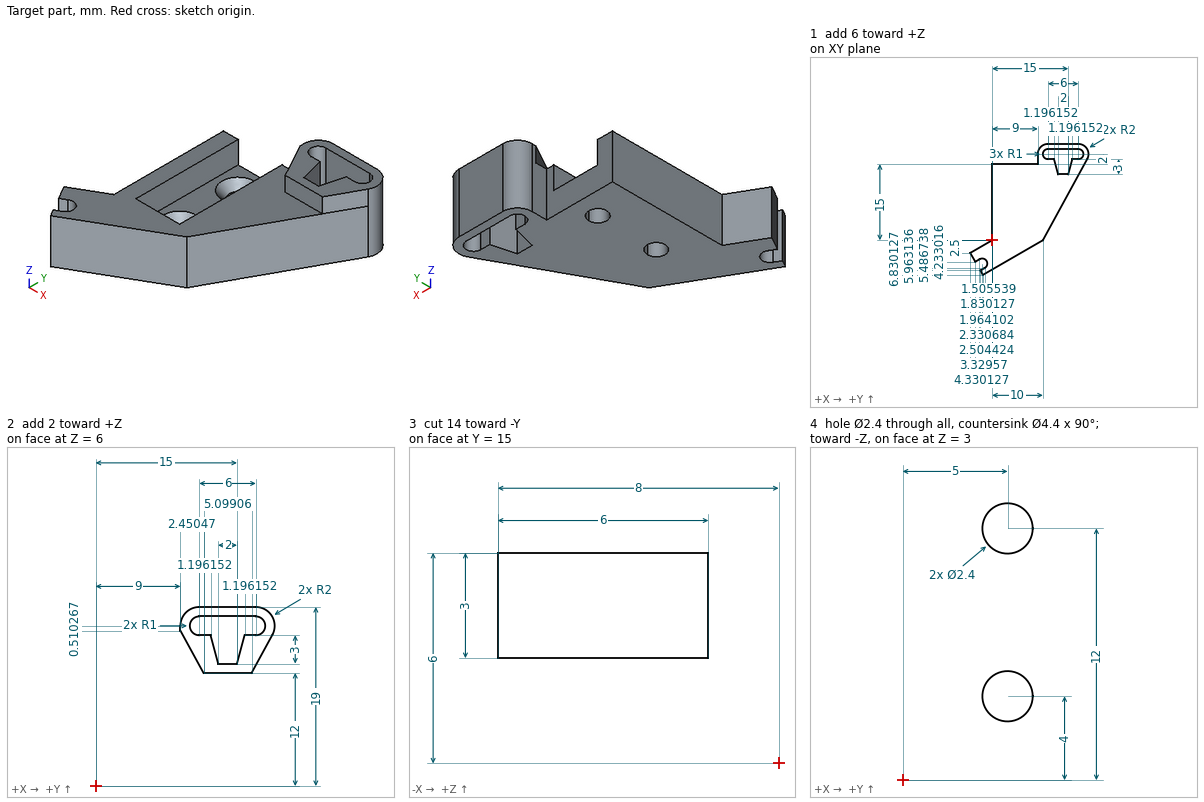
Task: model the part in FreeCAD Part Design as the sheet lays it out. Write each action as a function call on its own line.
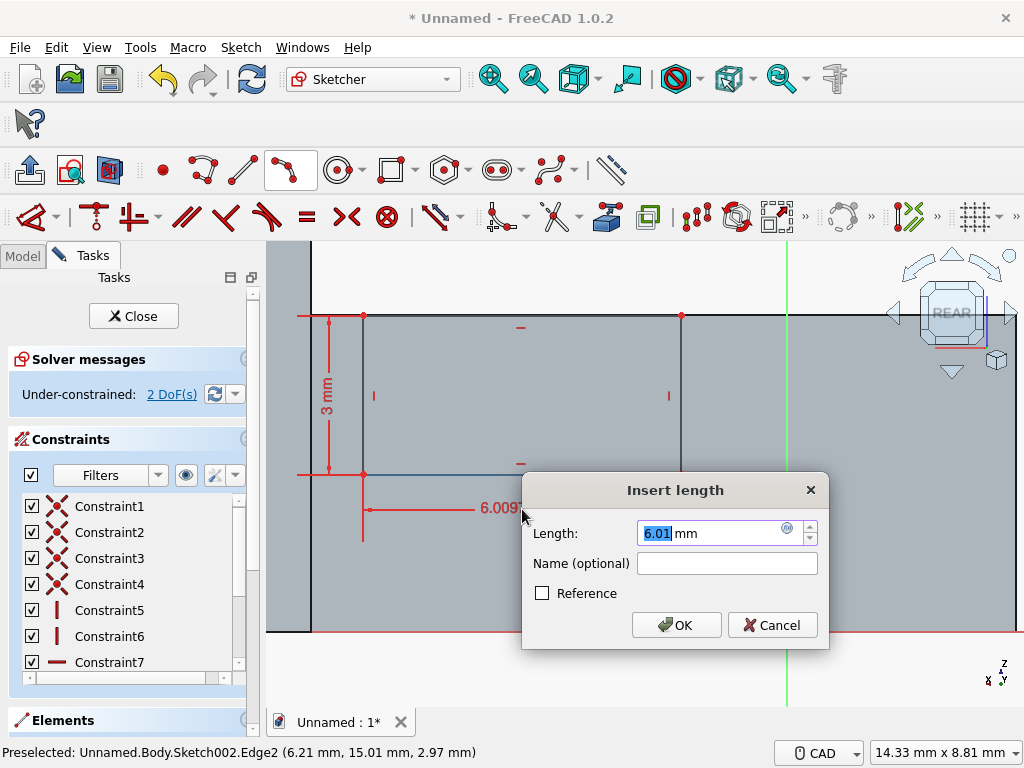
text(6)
key(Return)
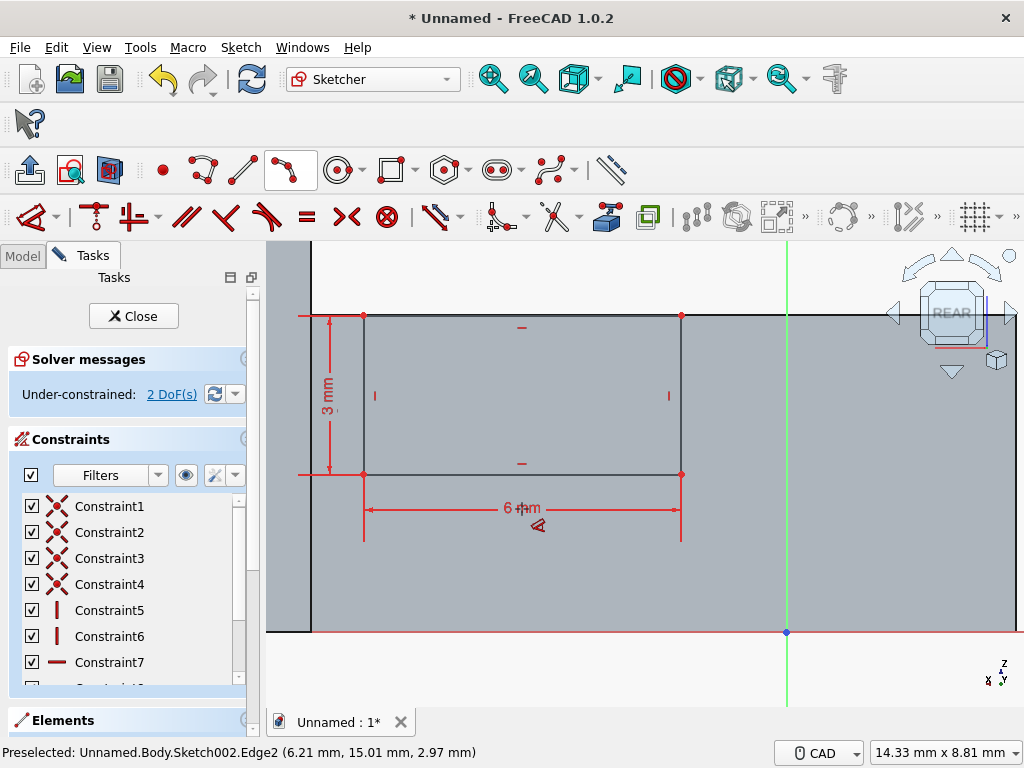
click(364, 316)
click(575, 666)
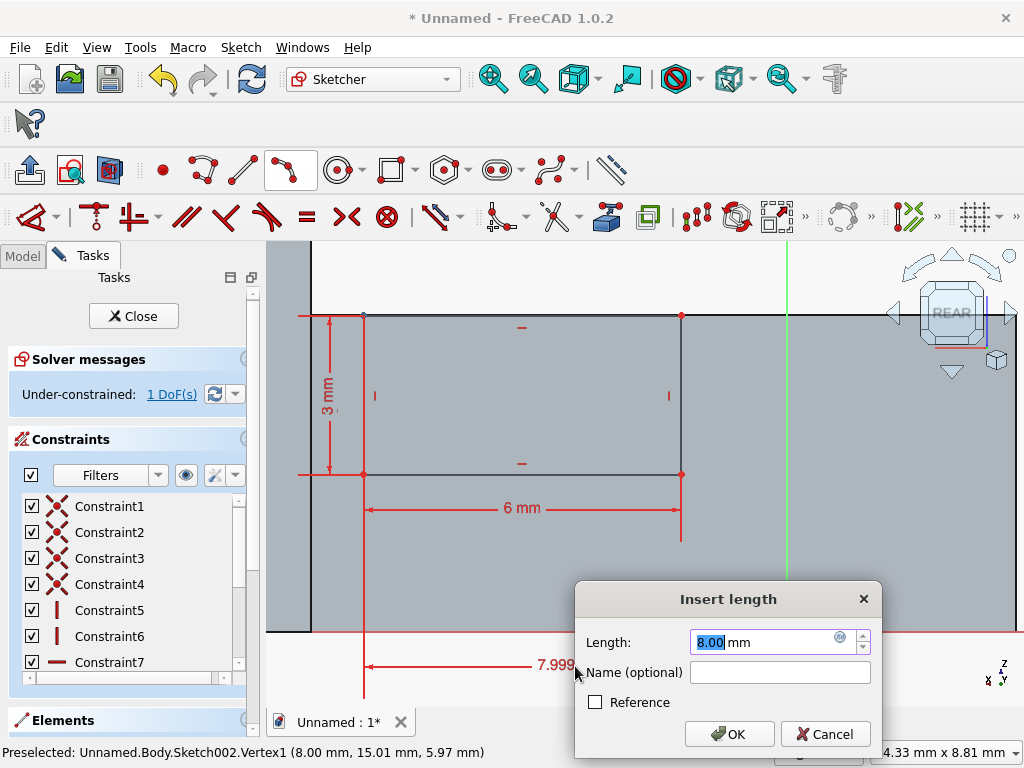
text(8)
key(Return)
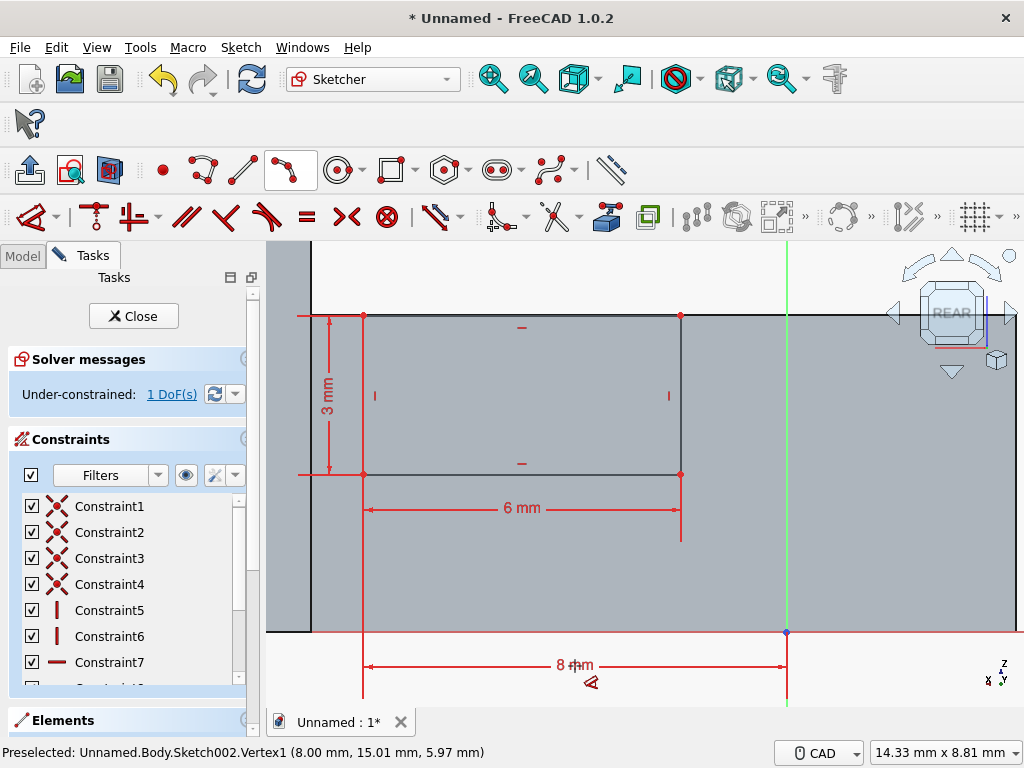
click(363, 316)
click(821, 474)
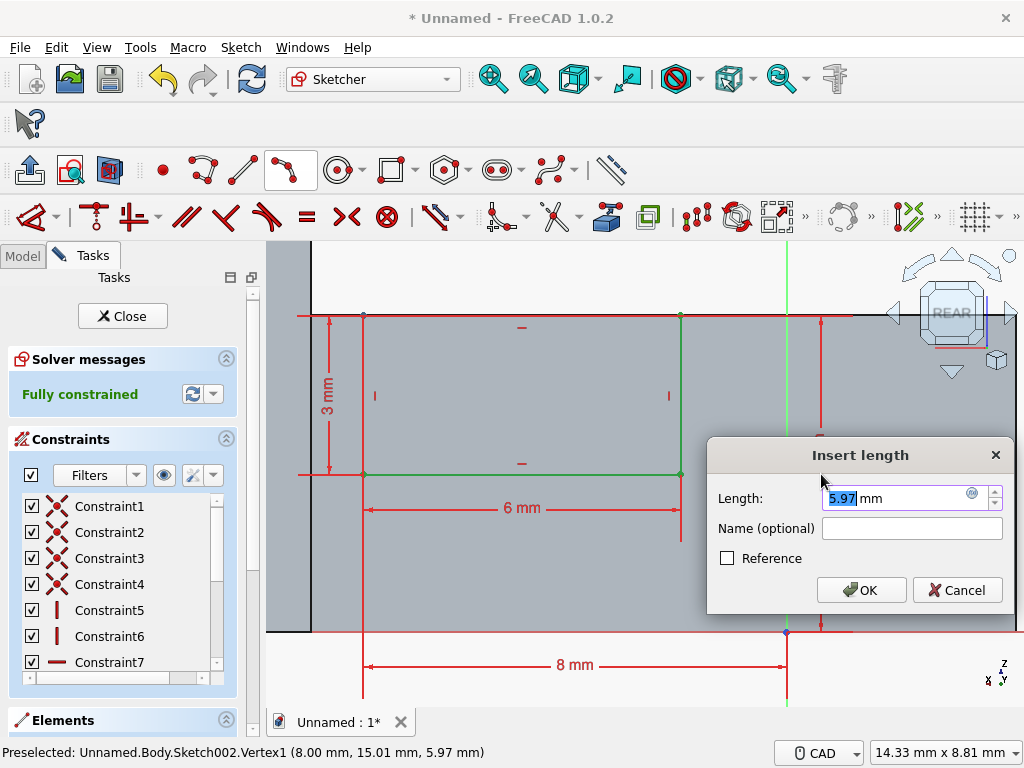
text(6)
key(Return)
key(Escape)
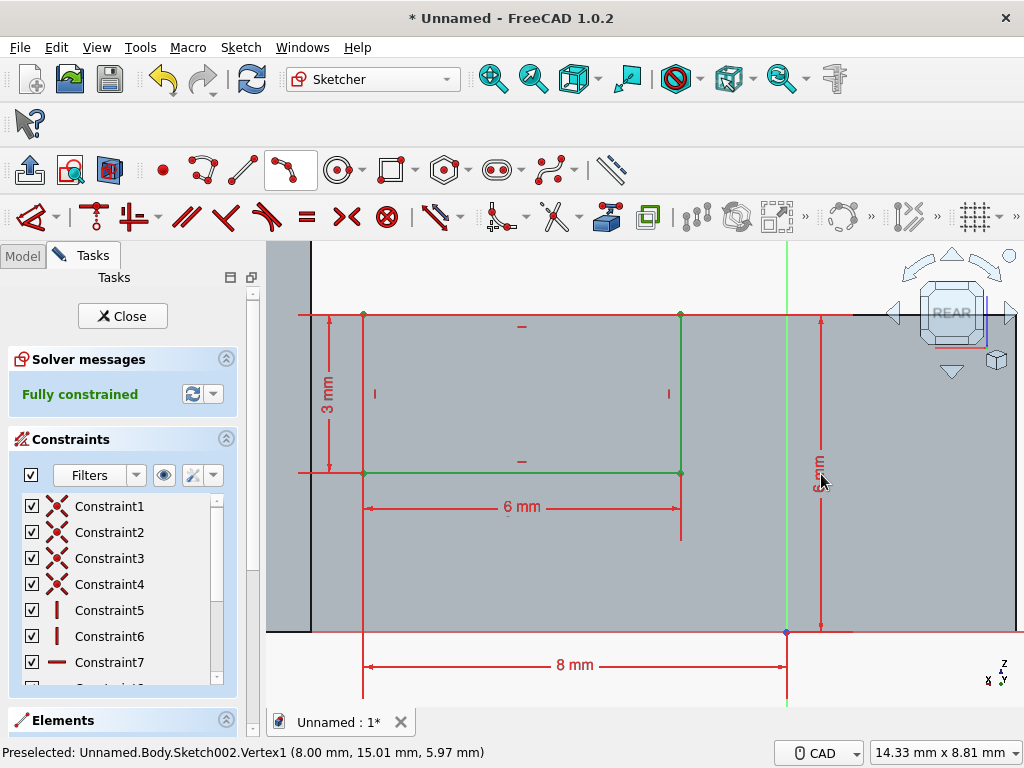
click(123, 316)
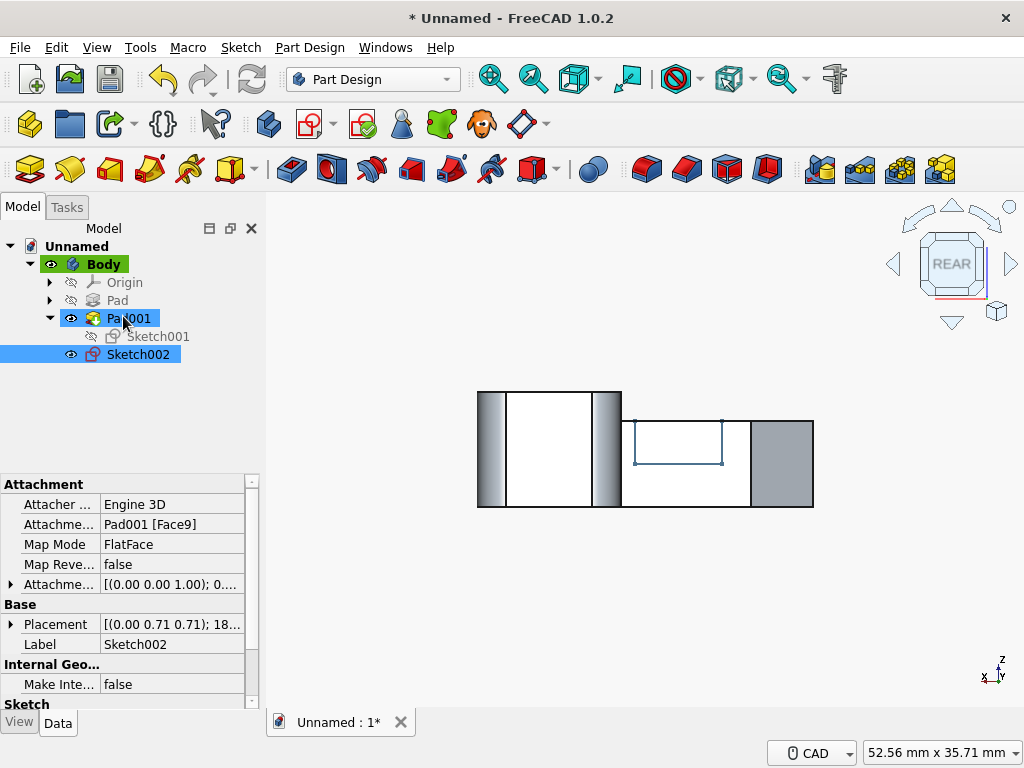
click(292, 170)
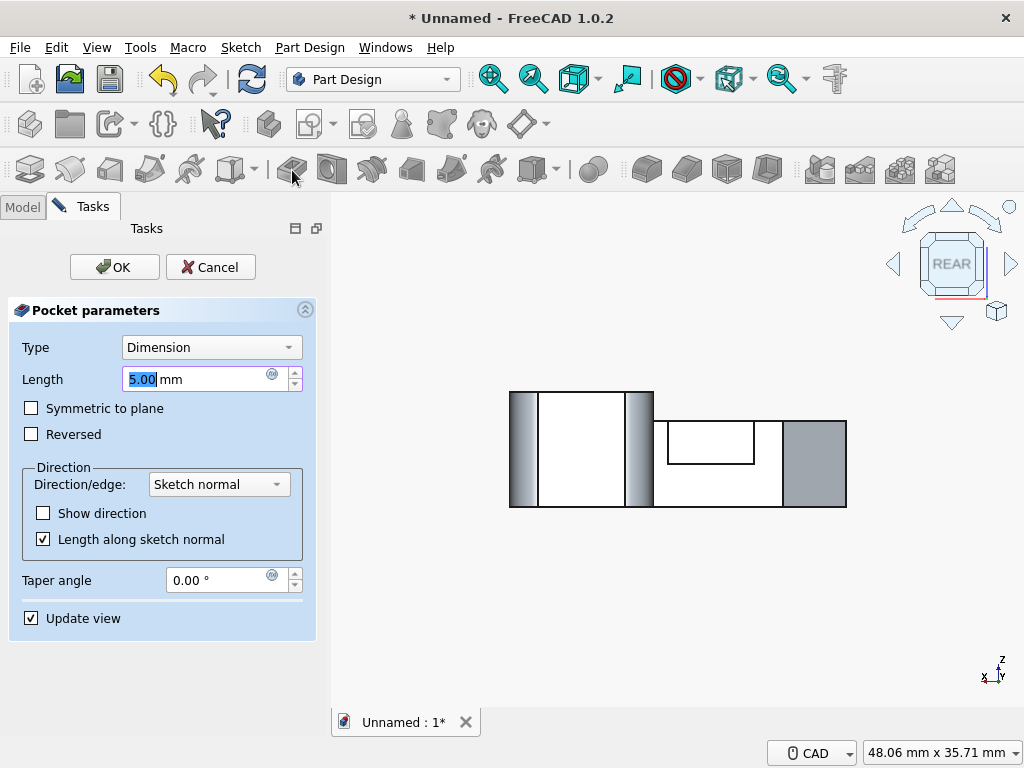
text(14)
key(Tab)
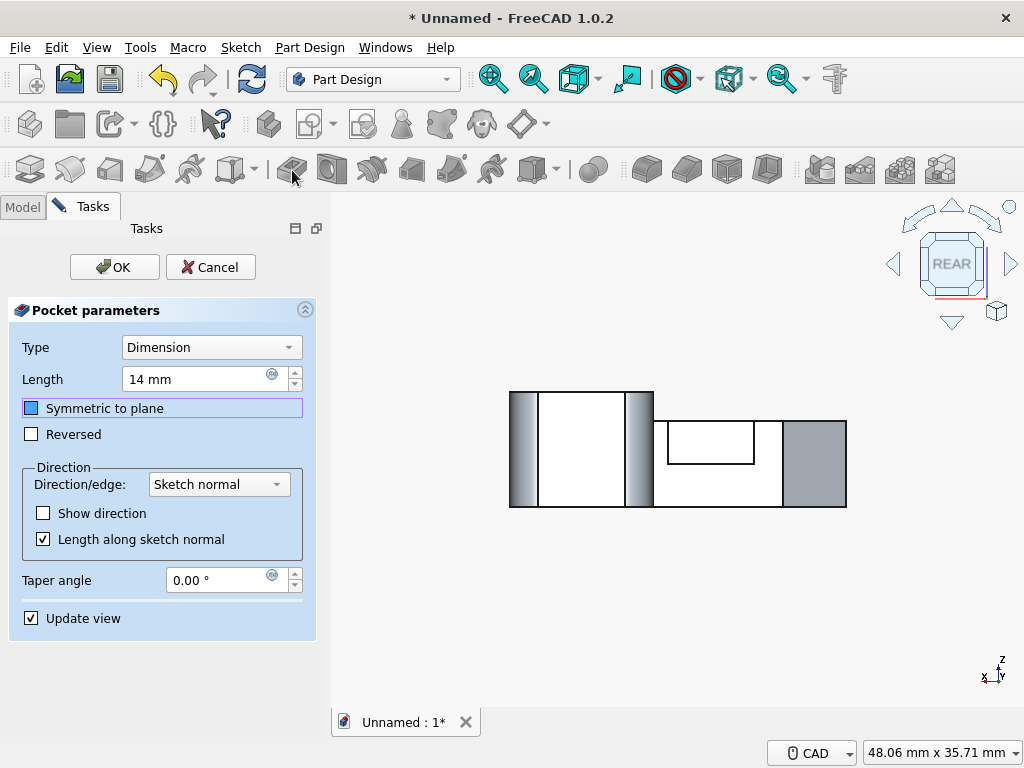
click(115, 267)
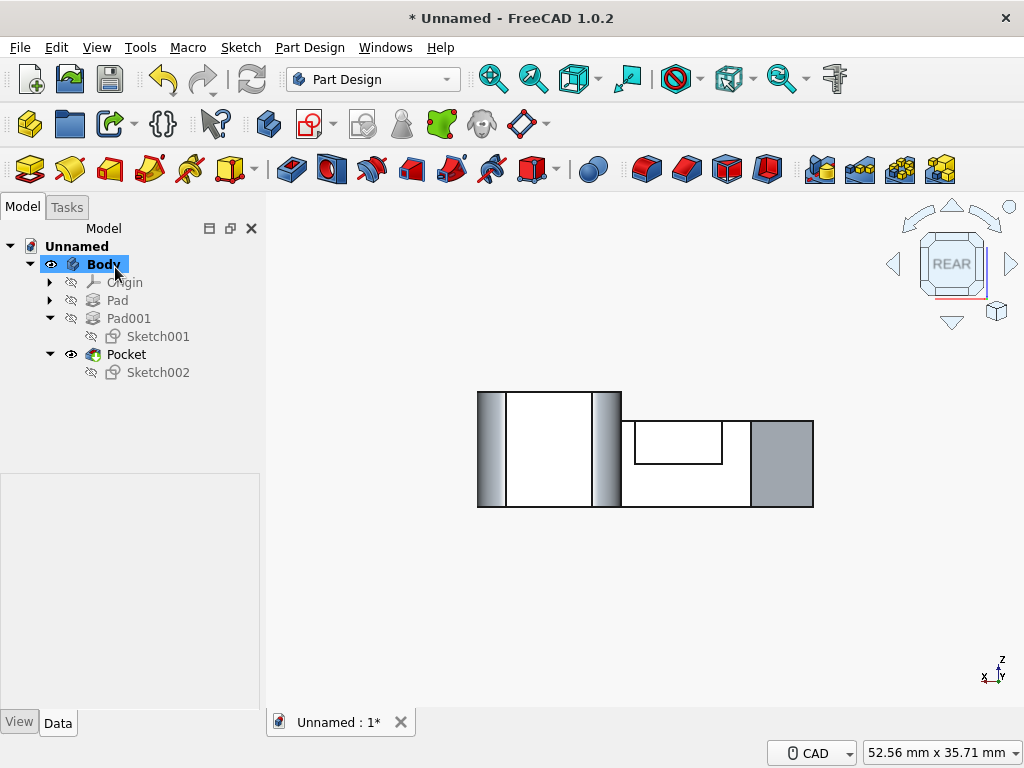
key(v)
key(f)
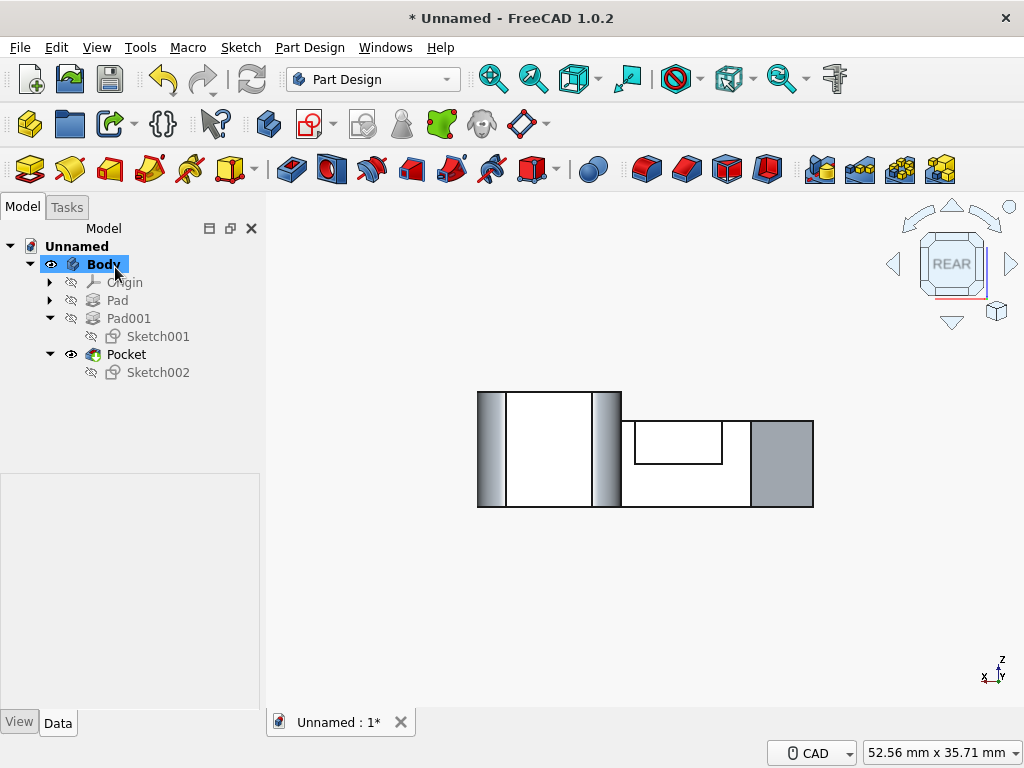
key(0)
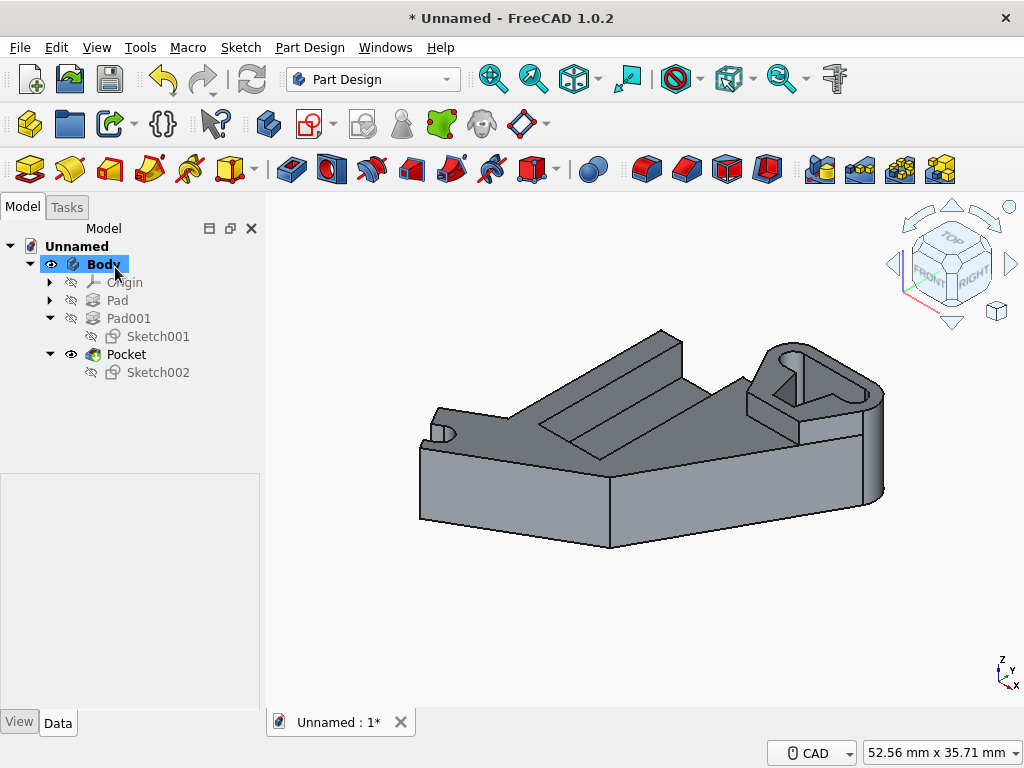
key(2)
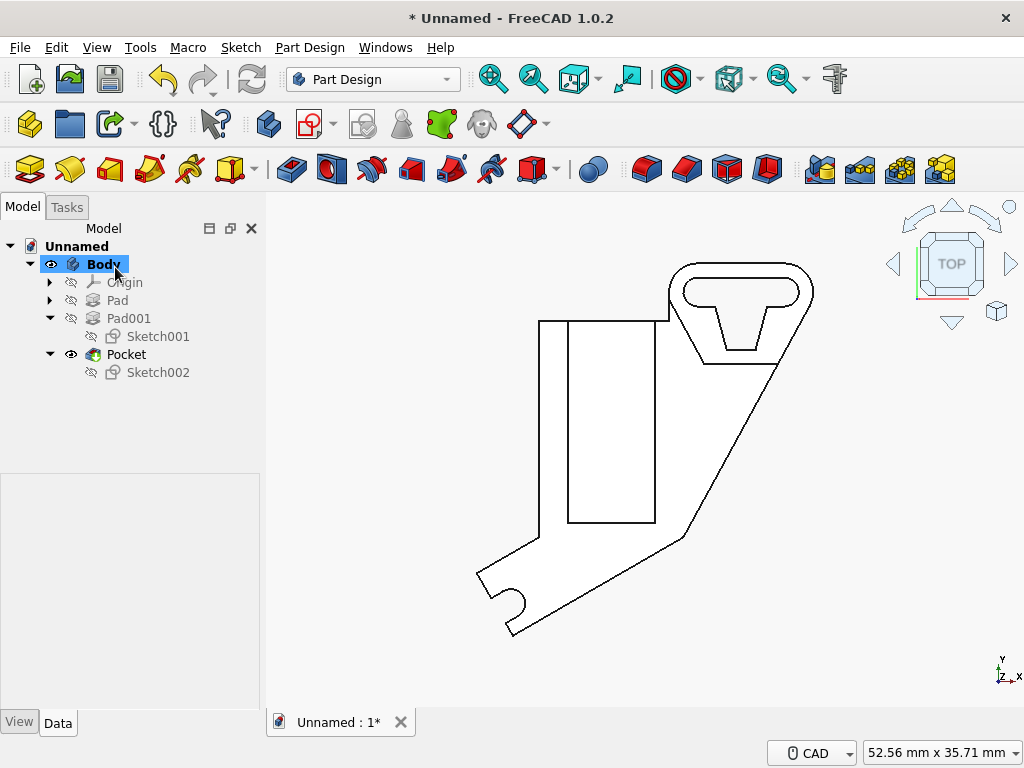
click(611, 363)